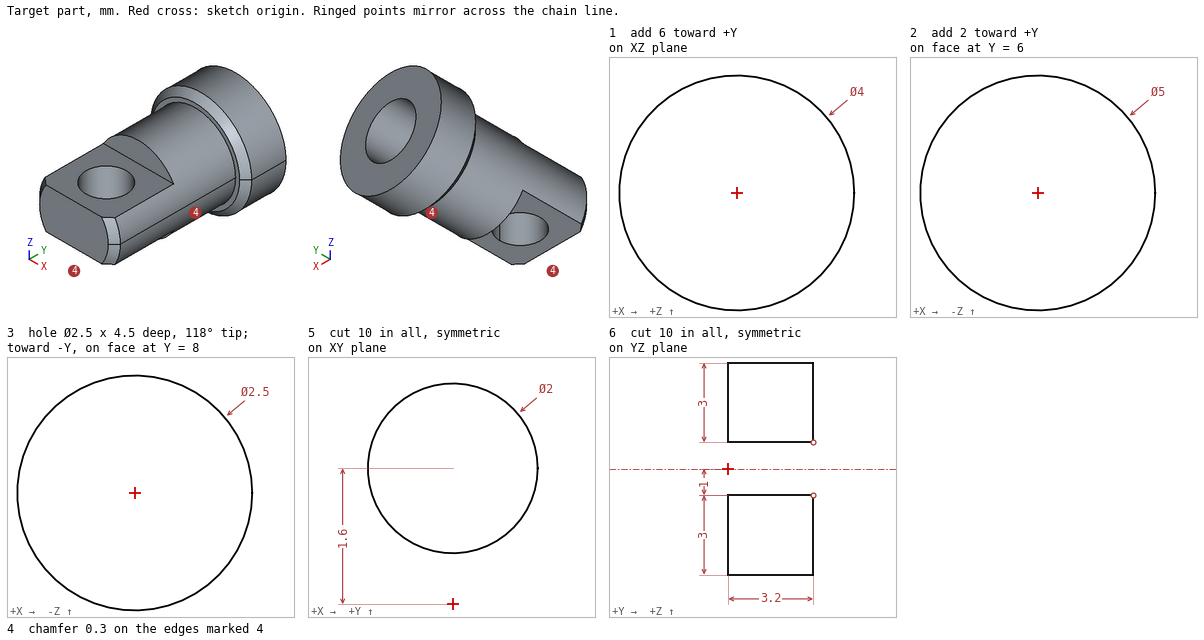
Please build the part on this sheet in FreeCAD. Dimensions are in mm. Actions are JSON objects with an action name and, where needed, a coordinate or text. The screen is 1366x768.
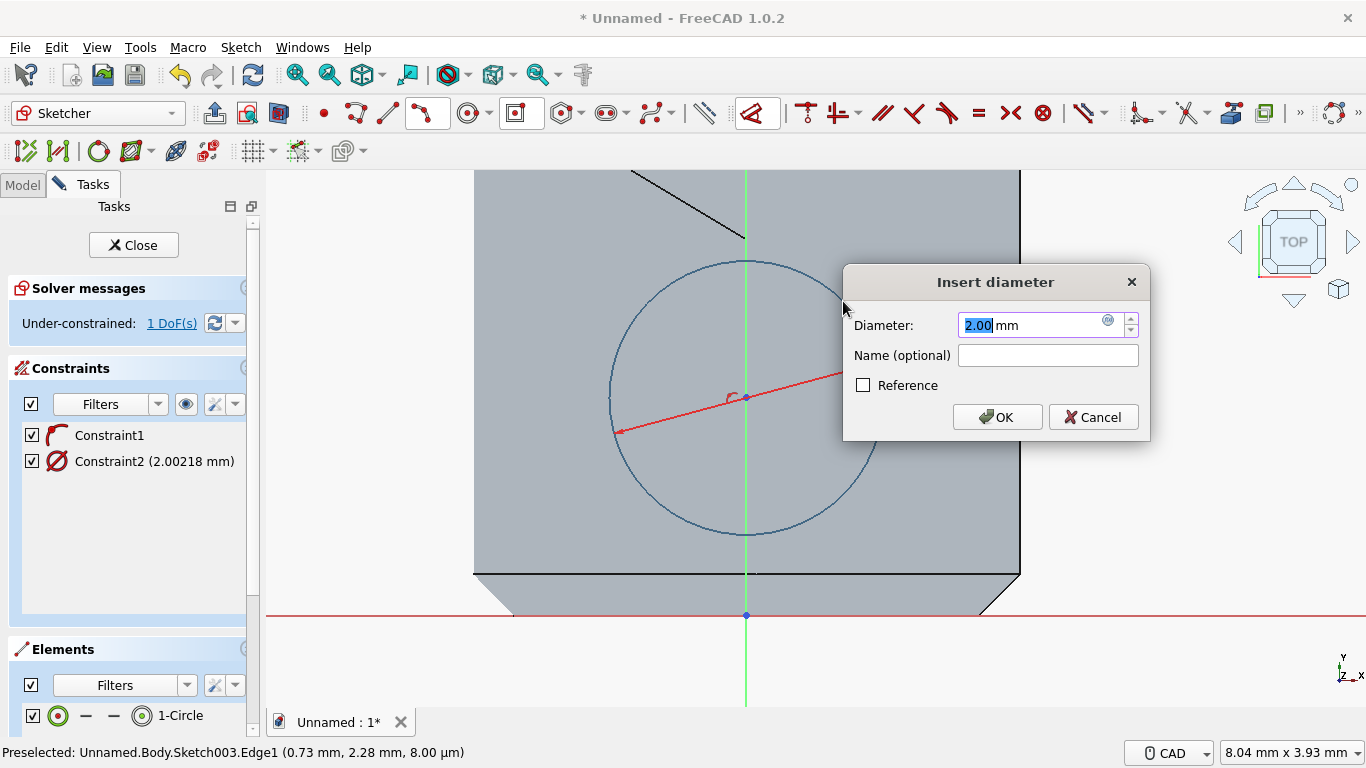
{"action": "type", "text": "2"}
{"action": "key", "text": "Return"}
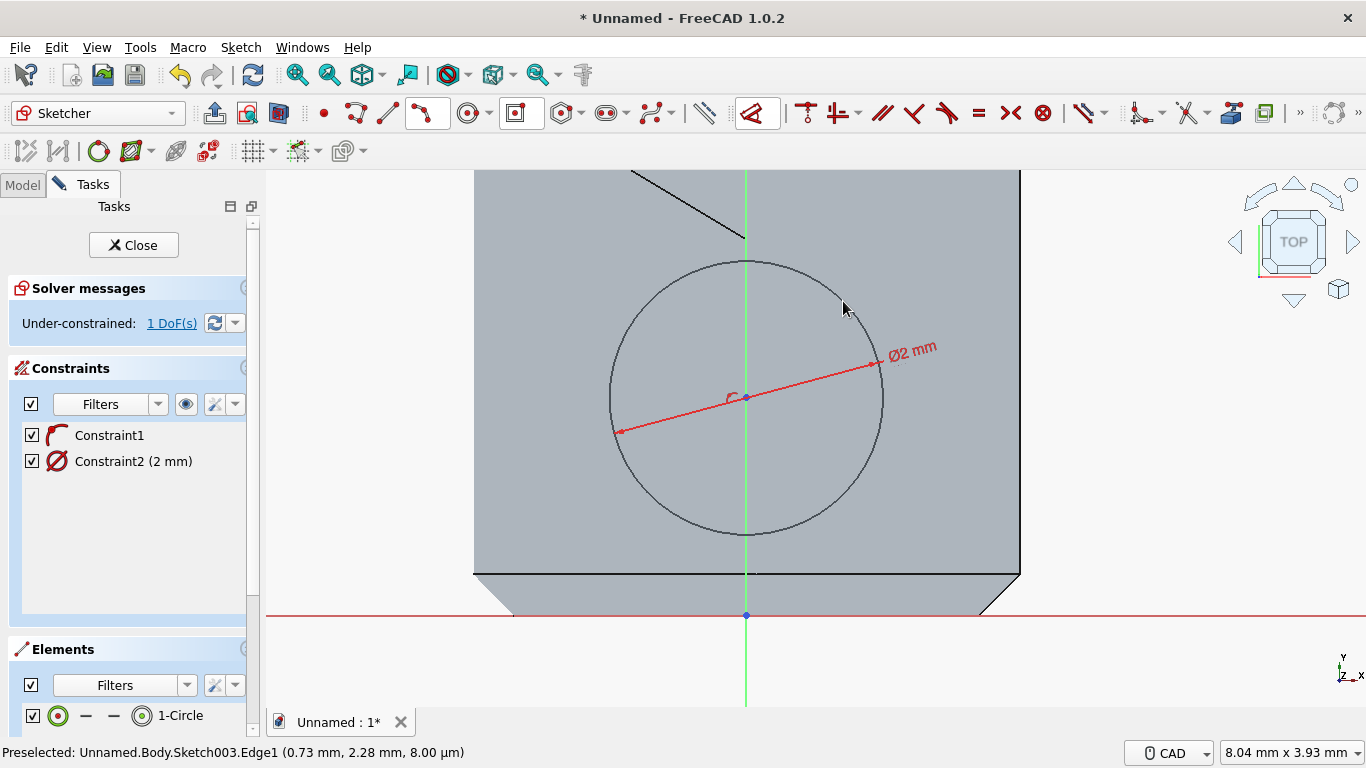
{"action": "left_click", "coordinate": [746, 398]}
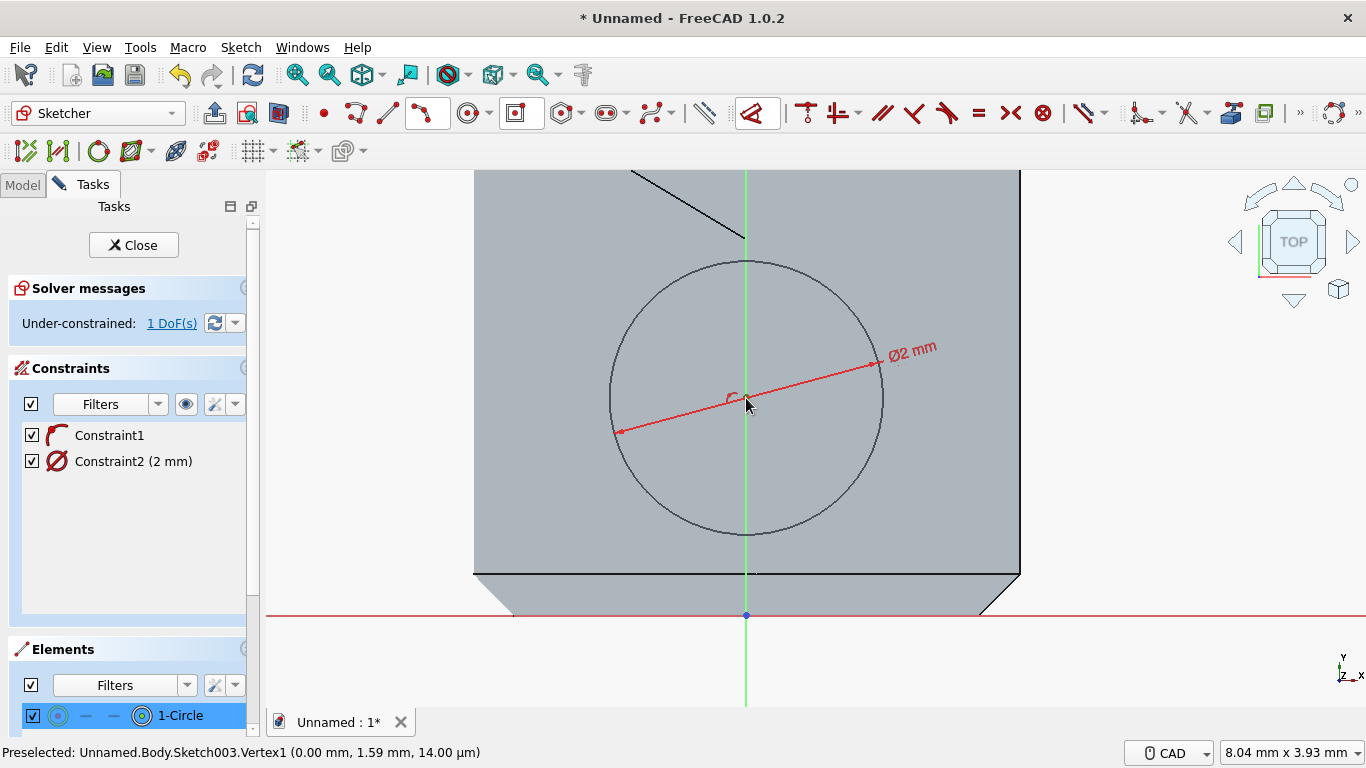
{"action": "key", "text": "i"}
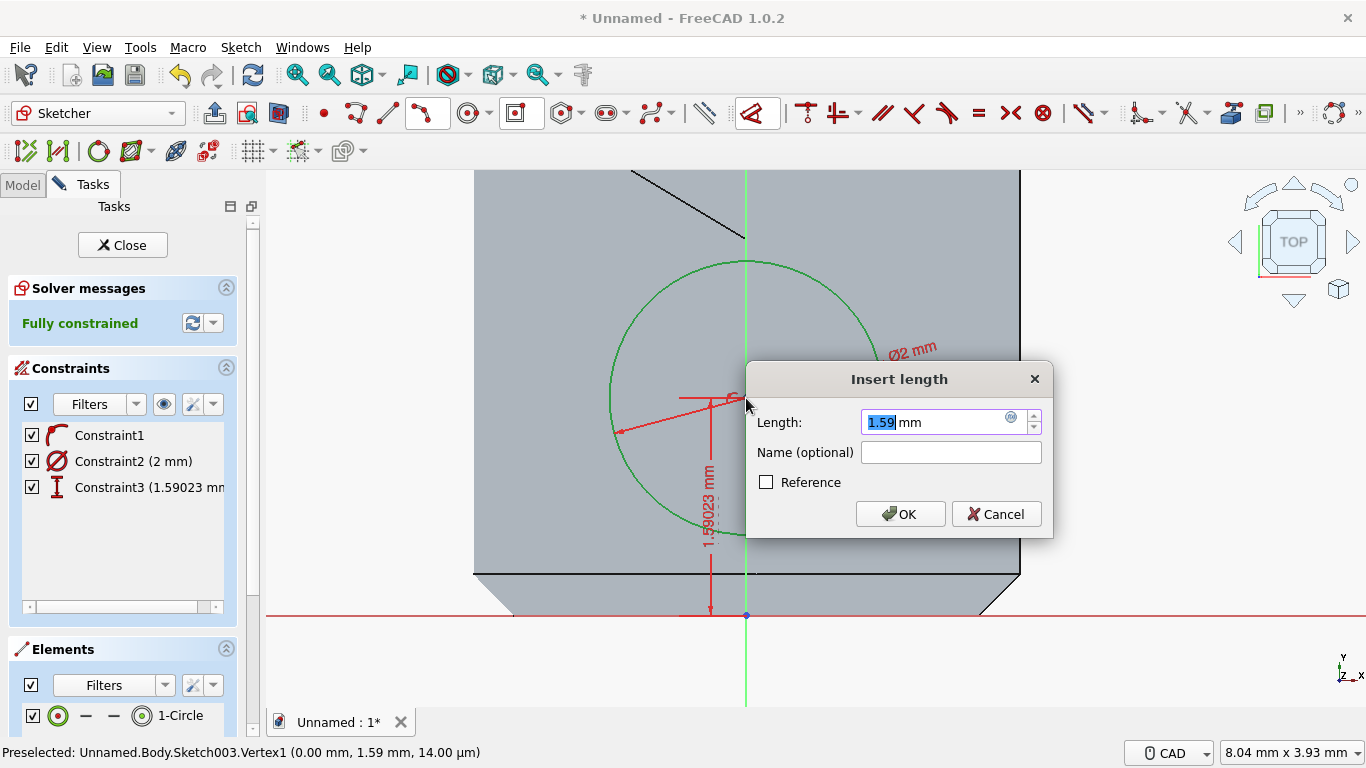
{"action": "type", "text": "1.6"}
{"action": "key", "text": "Return"}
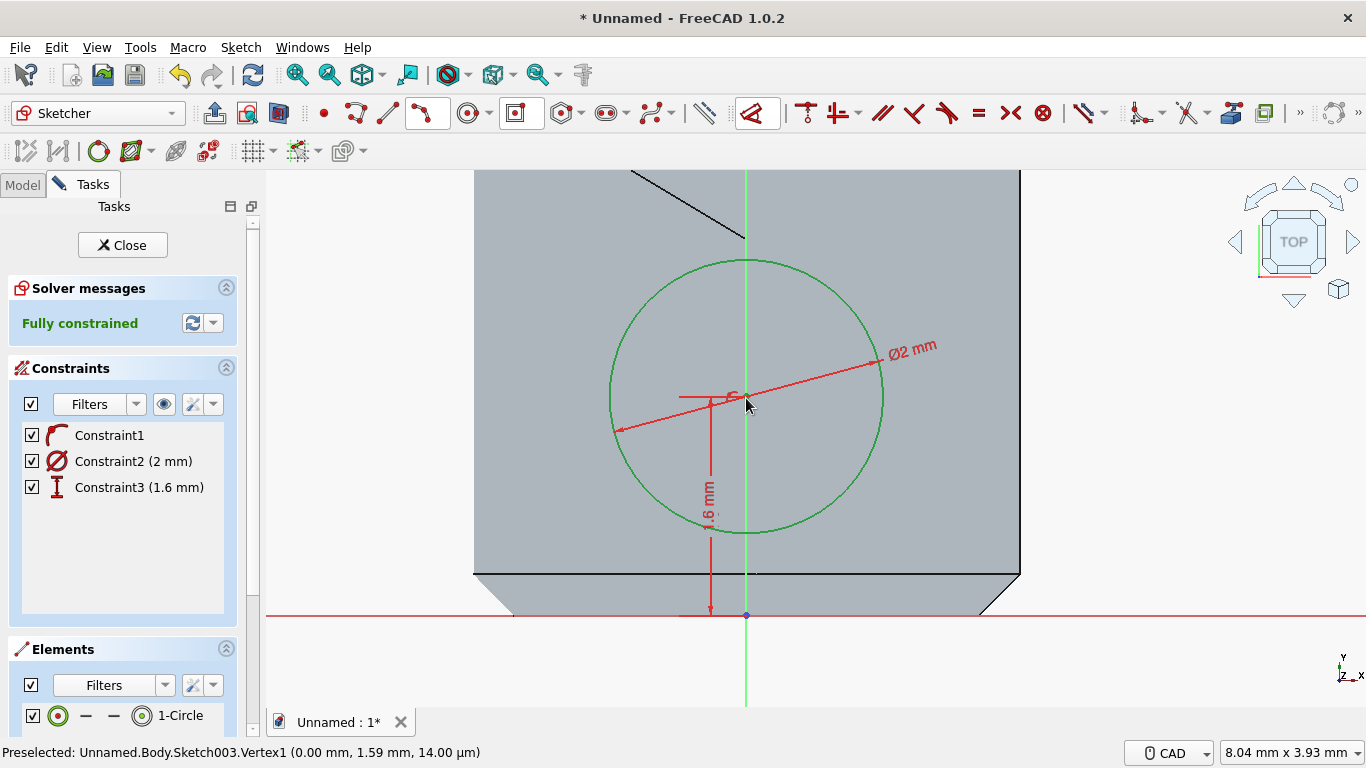
{"action": "left_click", "coordinate": [123, 245]}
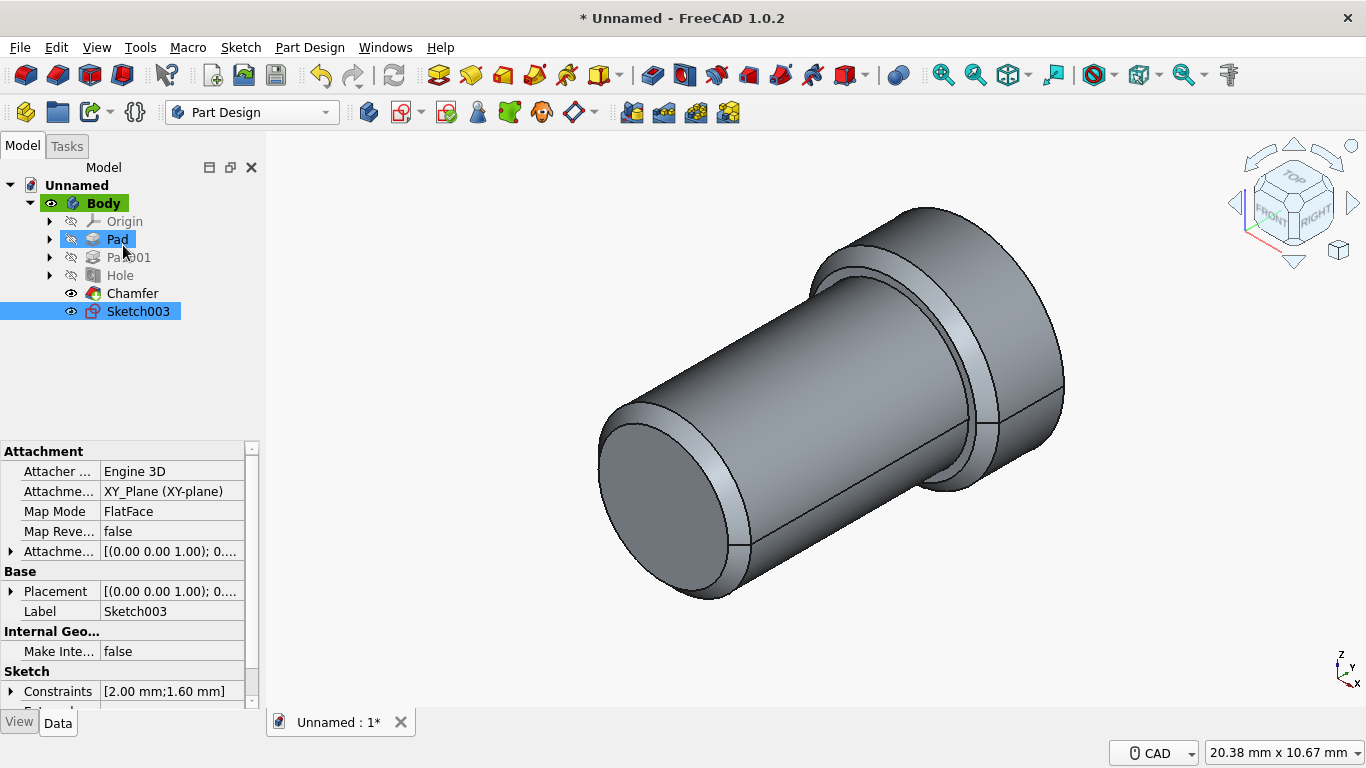
{"action": "left_click", "coordinate": [654, 76]}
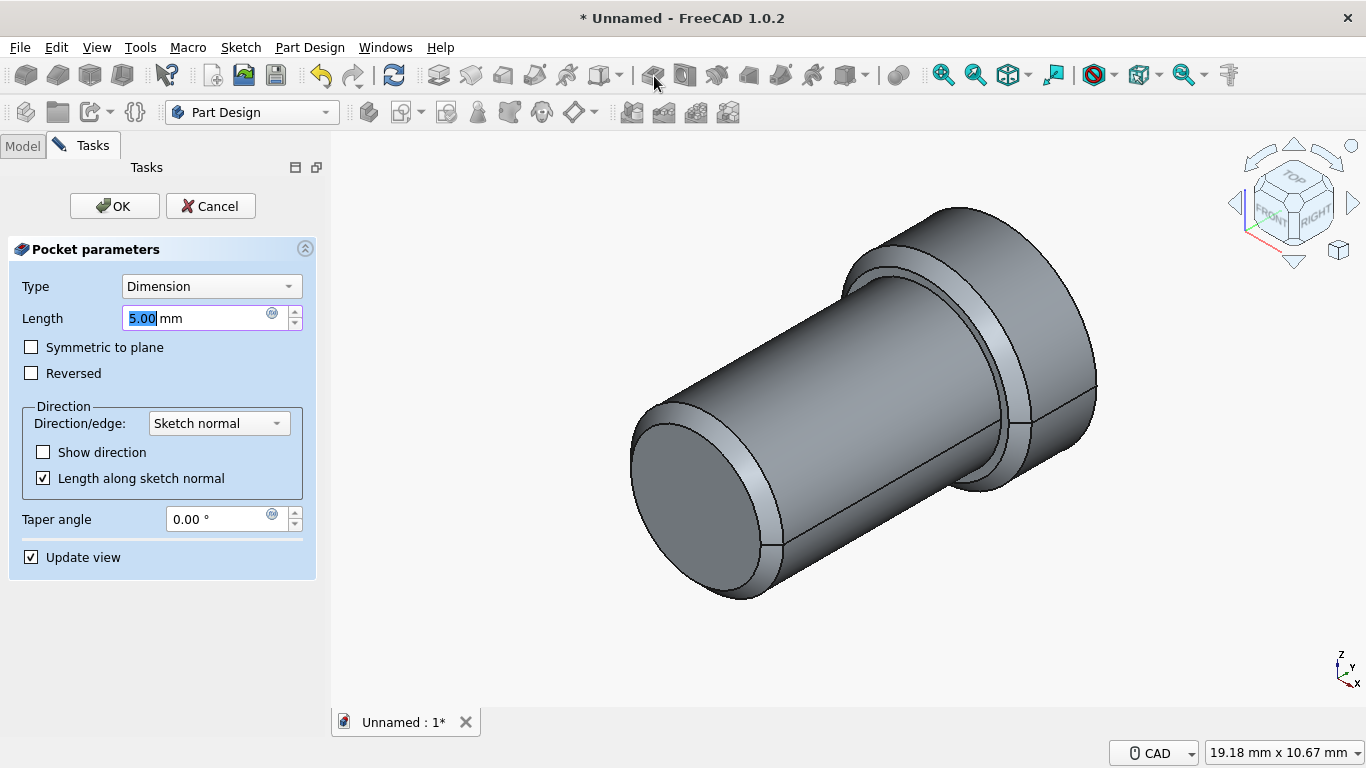
{"action": "type", "text": "10"}
{"action": "key", "text": "Tab"}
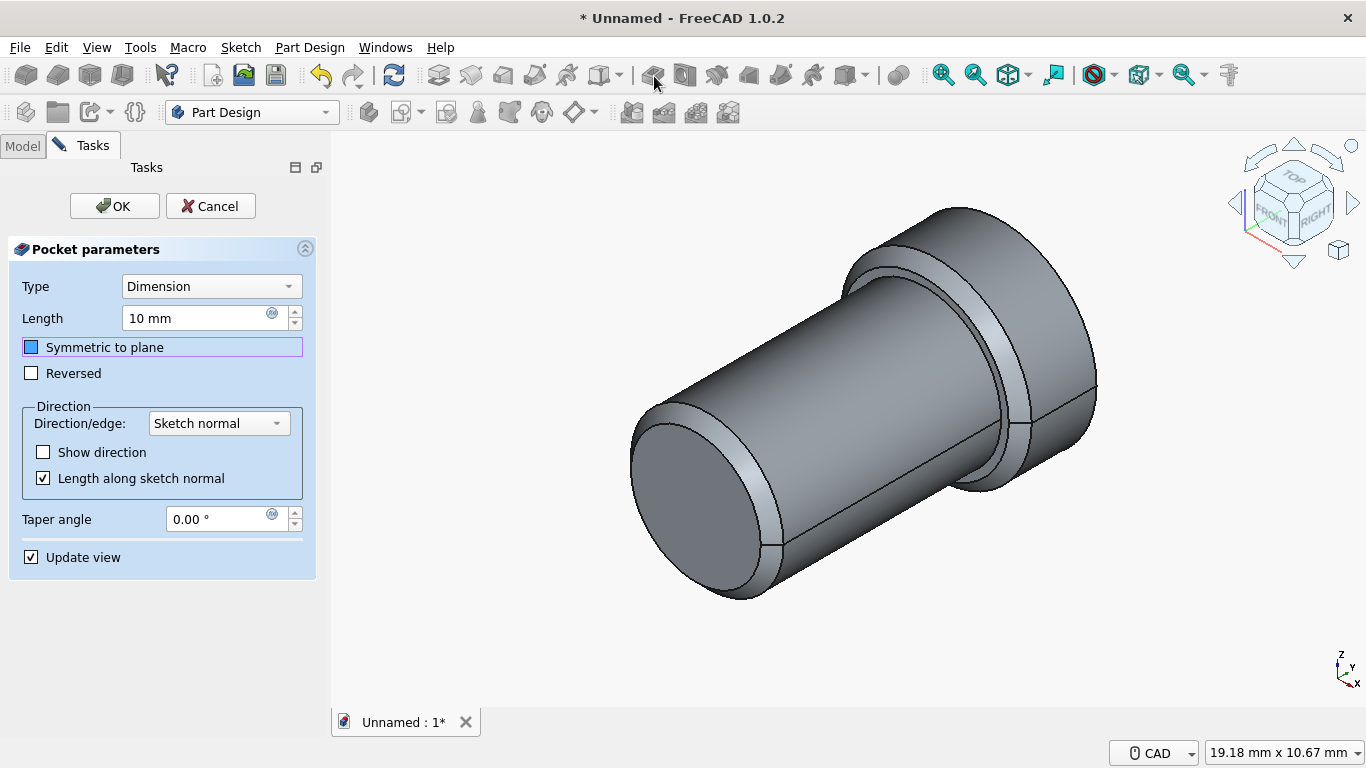
{"action": "left_click", "coordinate": [30, 347]}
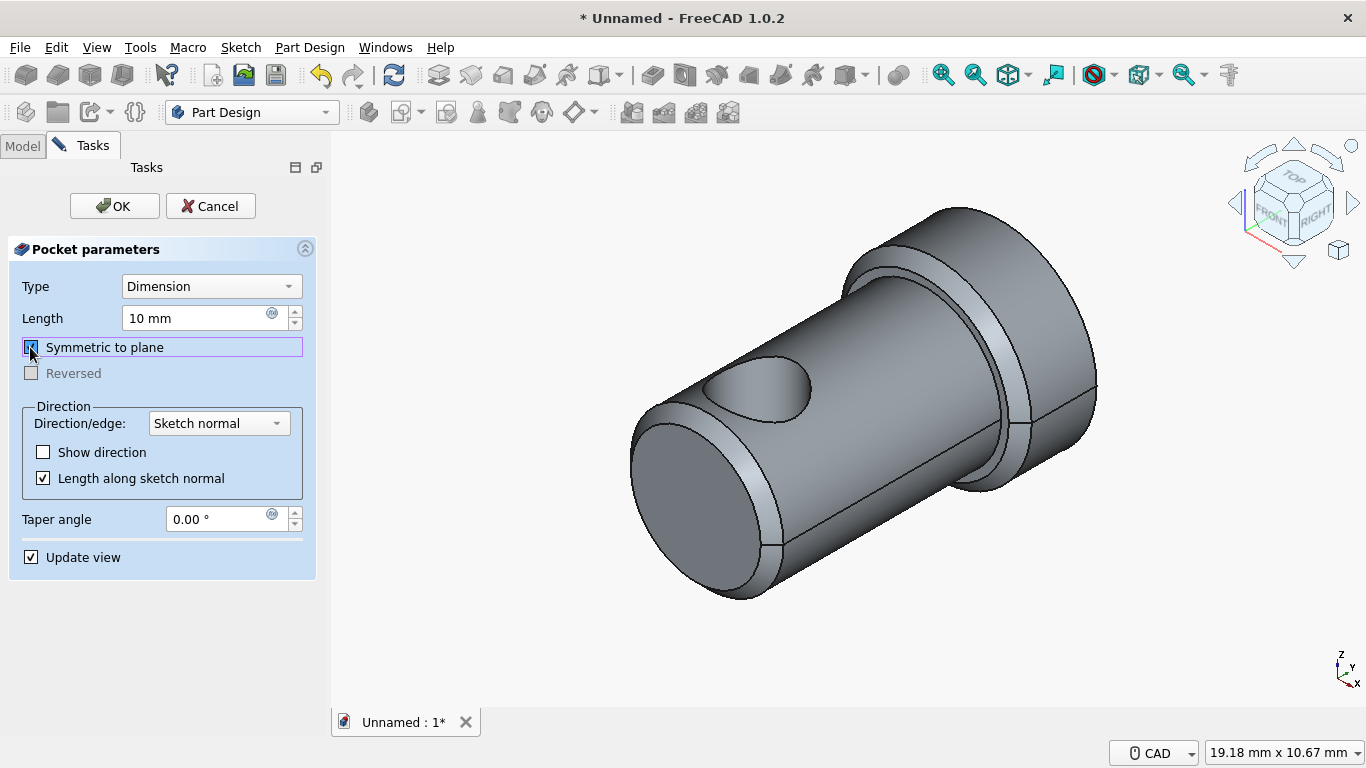
{"action": "left_click", "coordinate": [115, 206]}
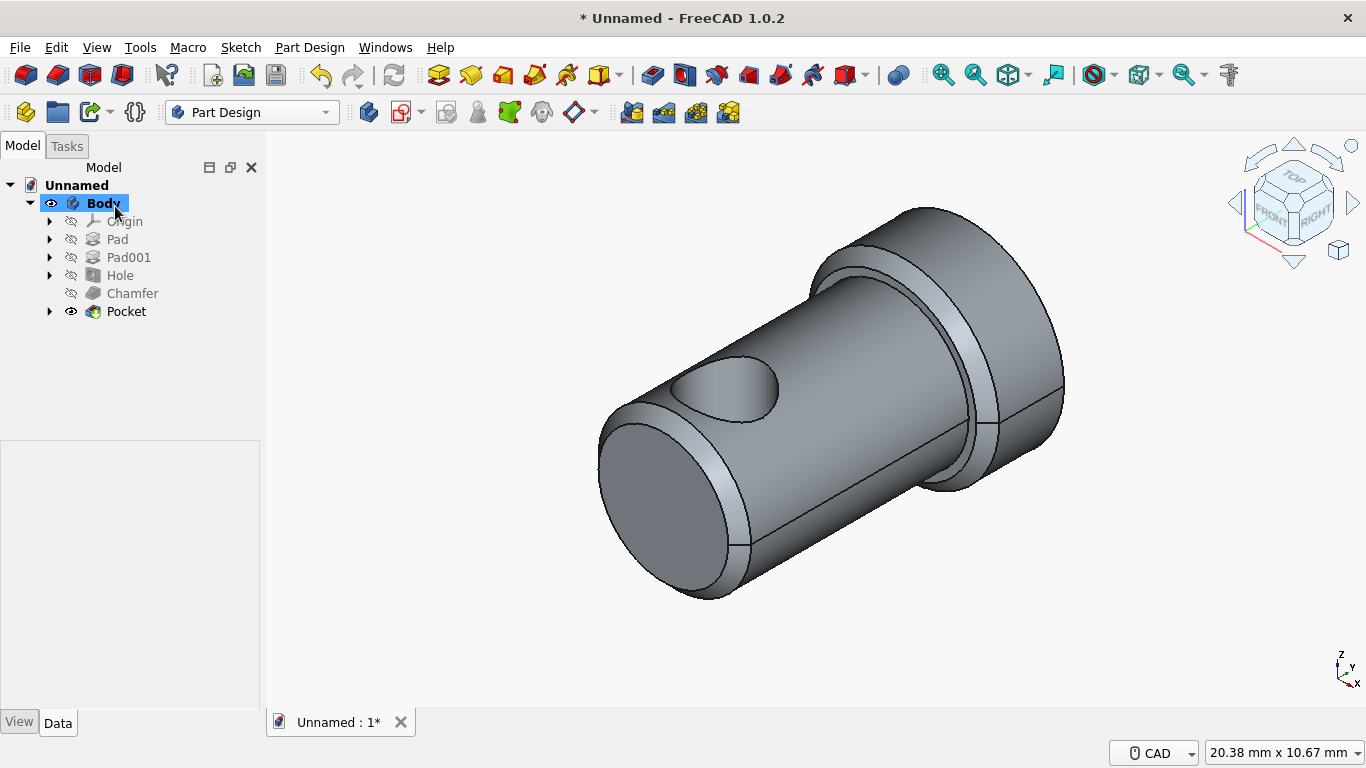
{"action": "left_click", "coordinate": [402, 112]}